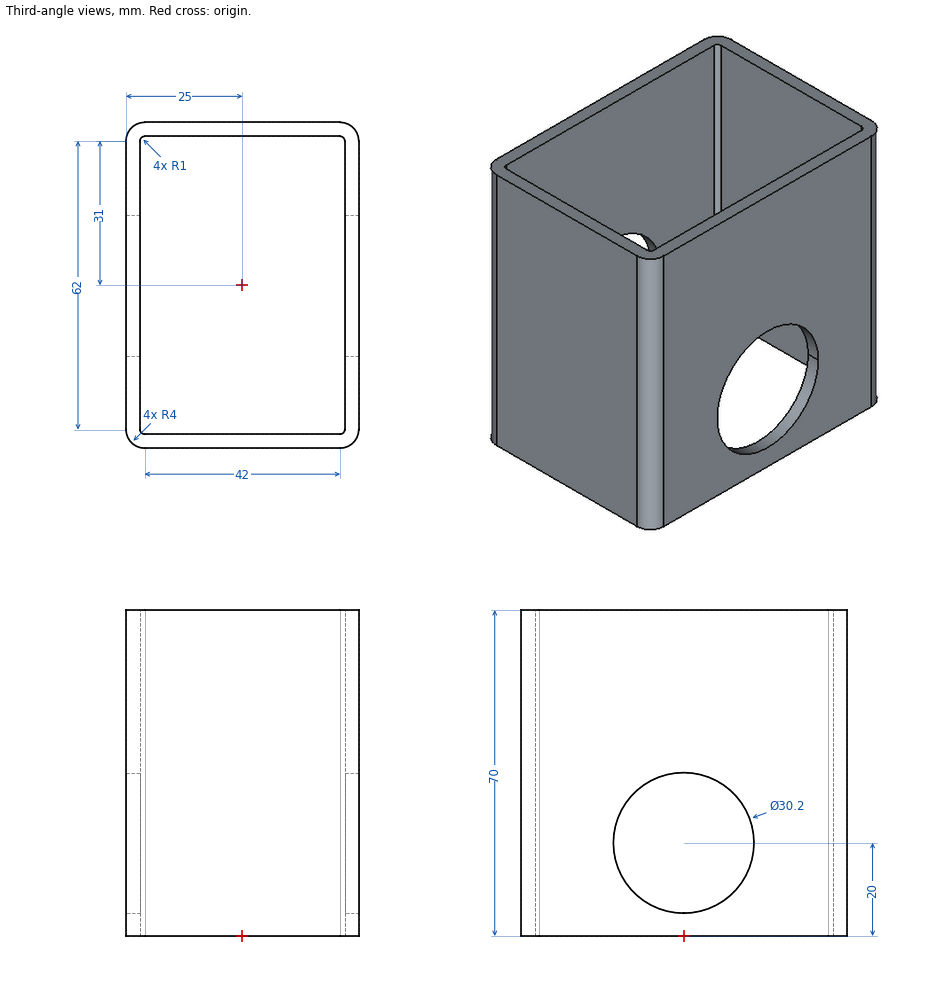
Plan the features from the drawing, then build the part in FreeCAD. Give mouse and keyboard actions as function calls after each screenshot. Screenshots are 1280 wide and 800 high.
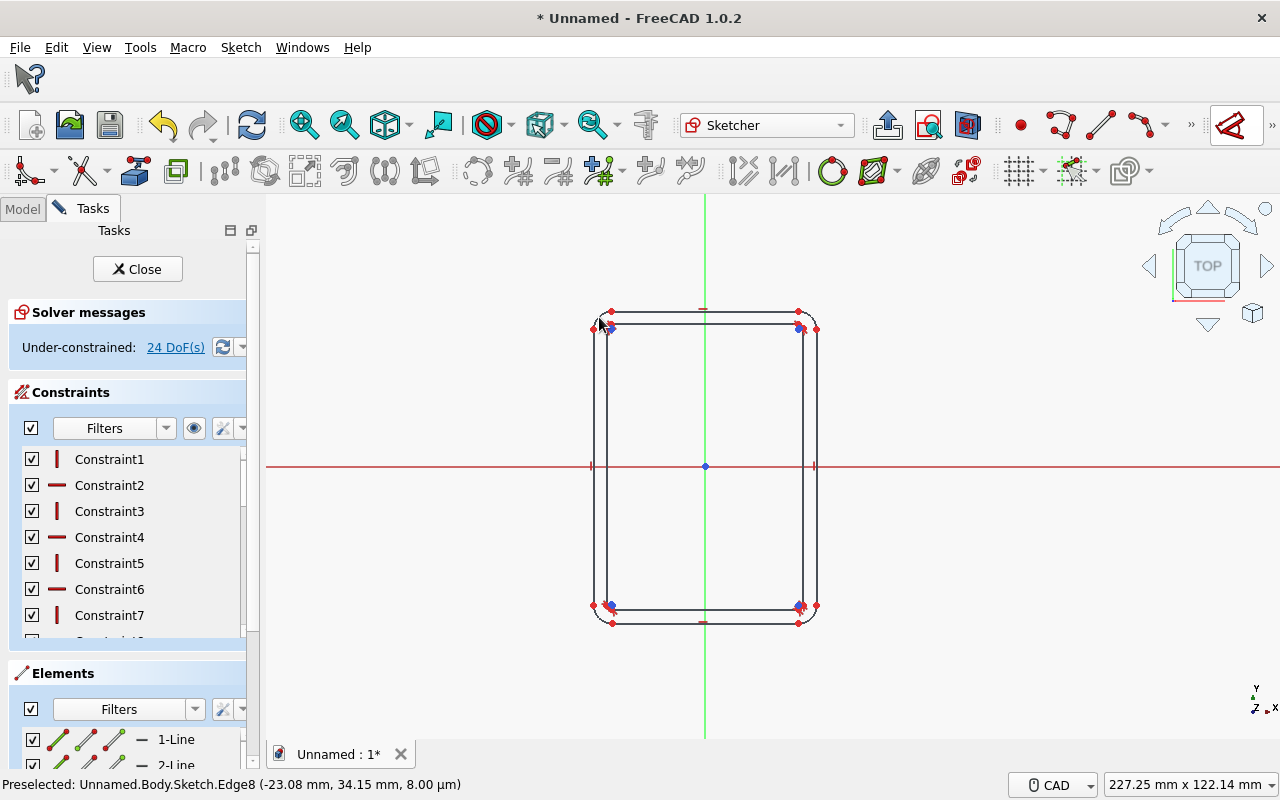
click(607, 522)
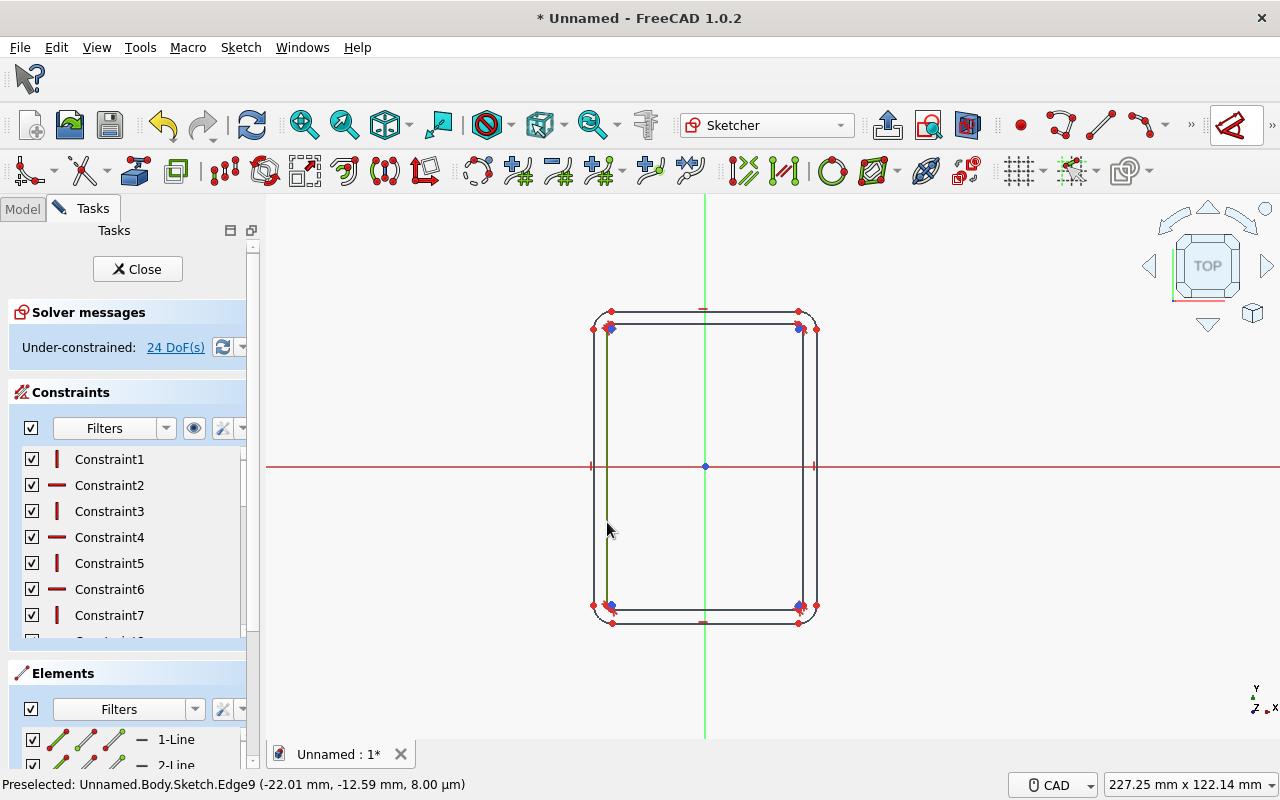
scroll(608, 326, up, 7)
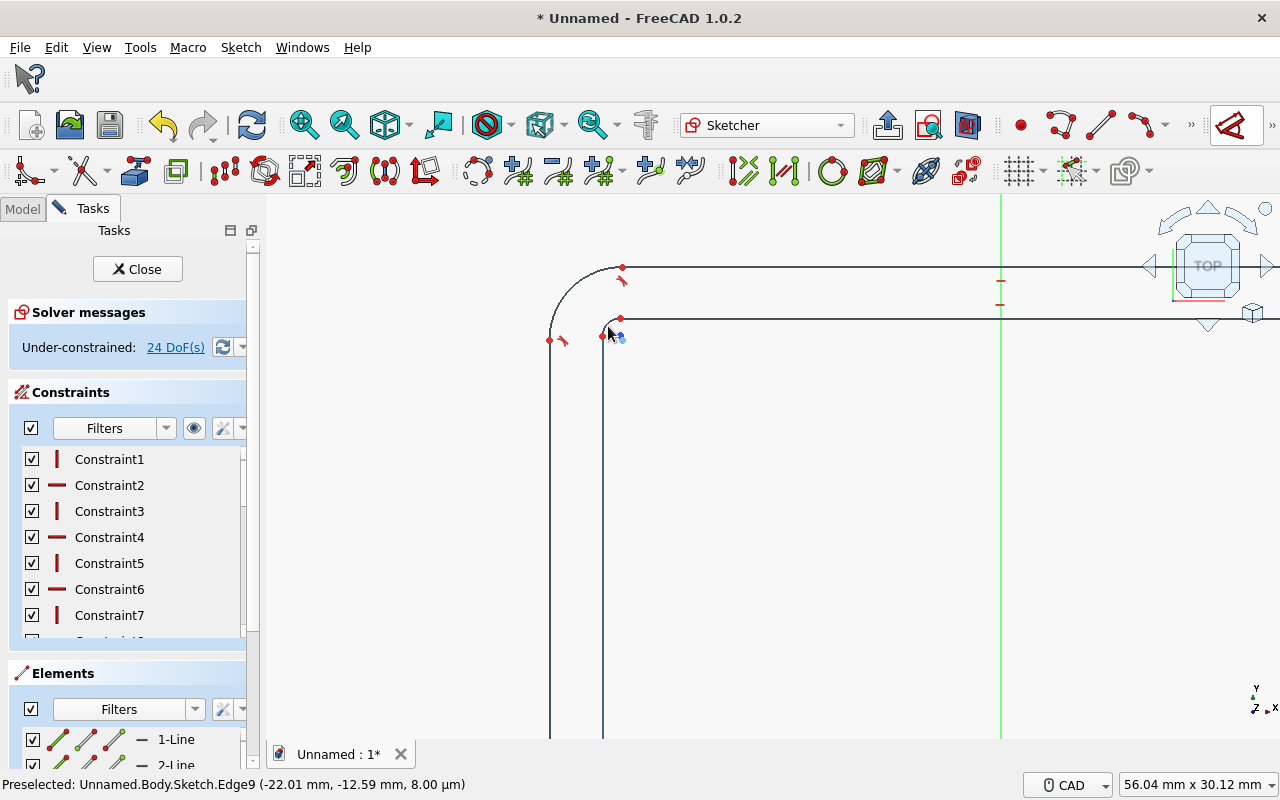
click(608, 324)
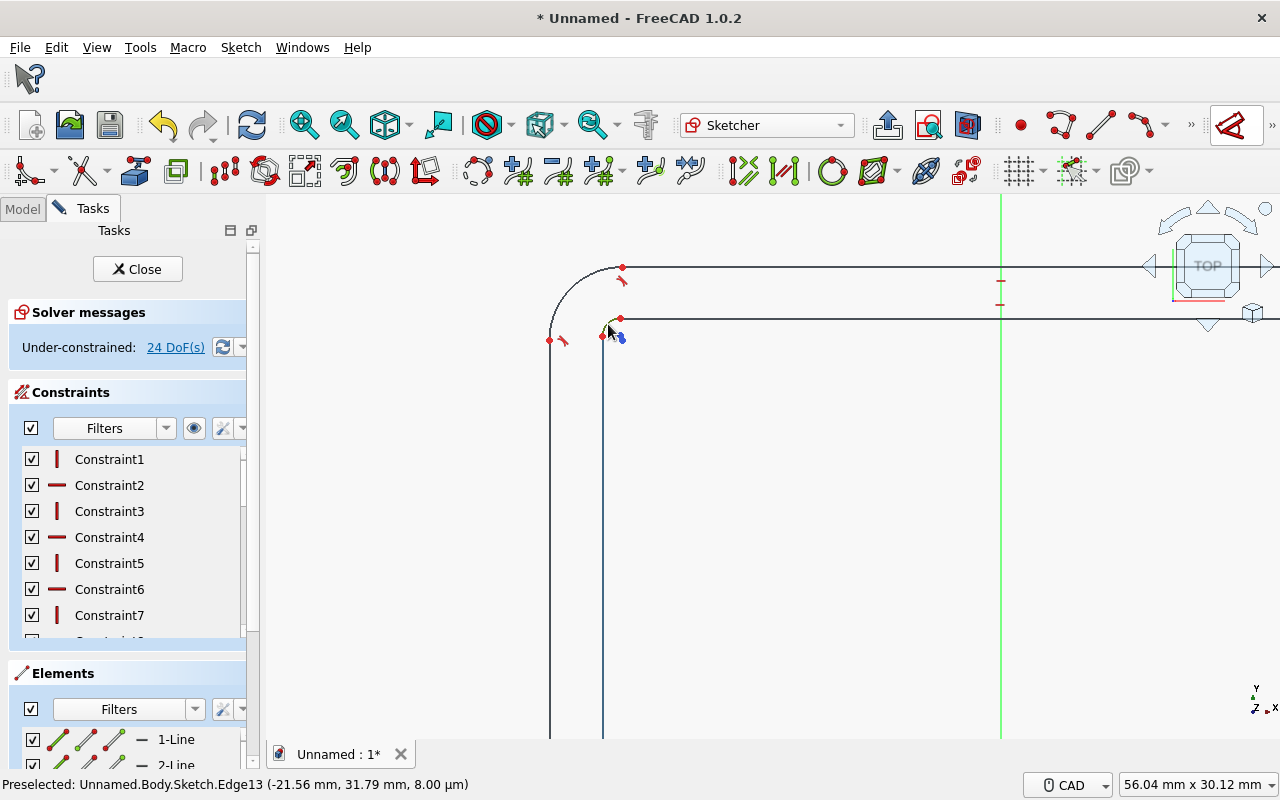
key(t)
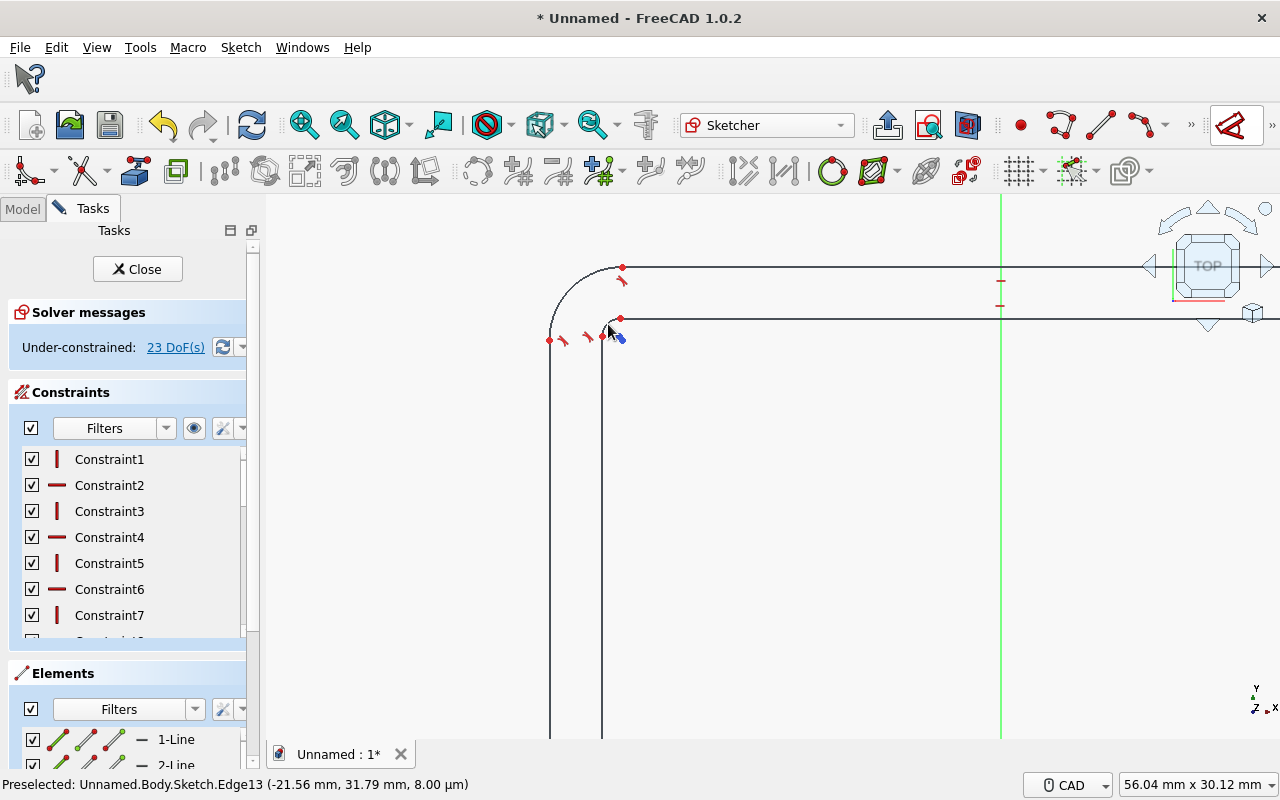
click(602, 673)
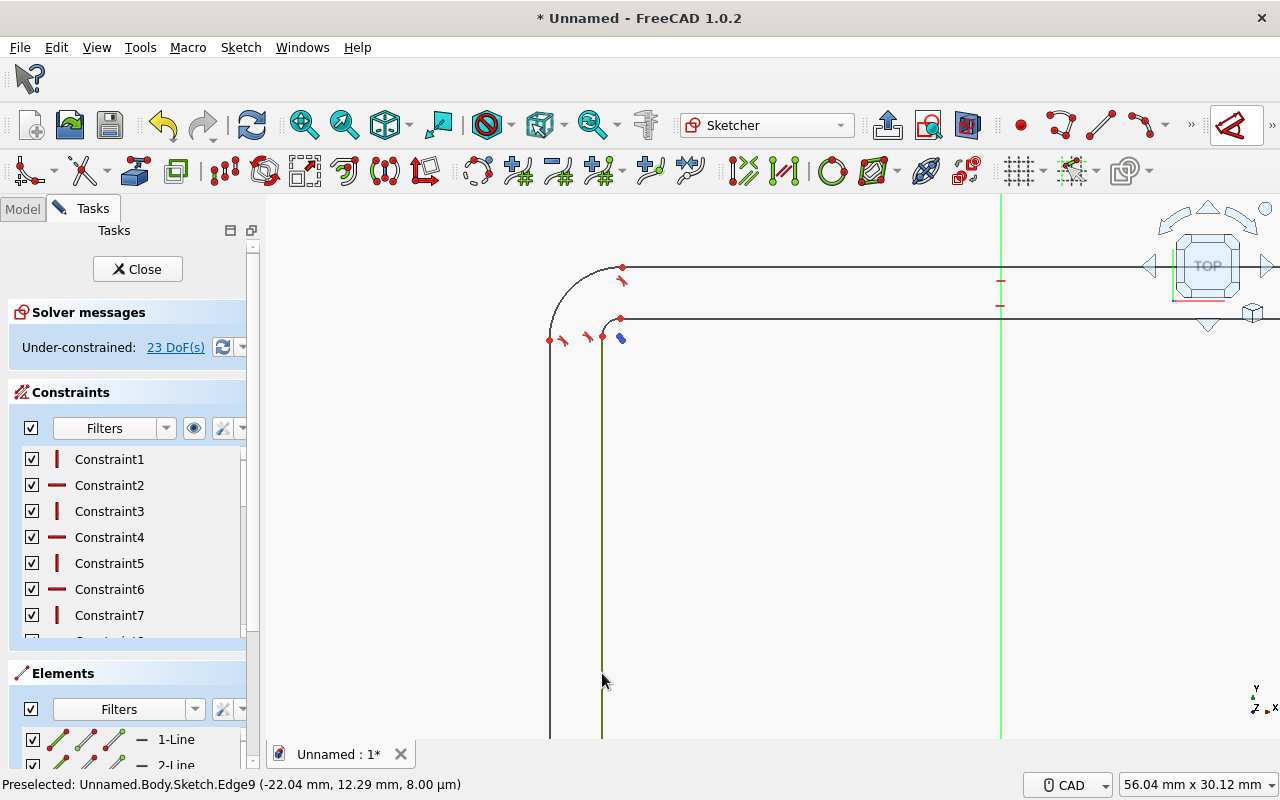
scroll(607, 326, down, 7)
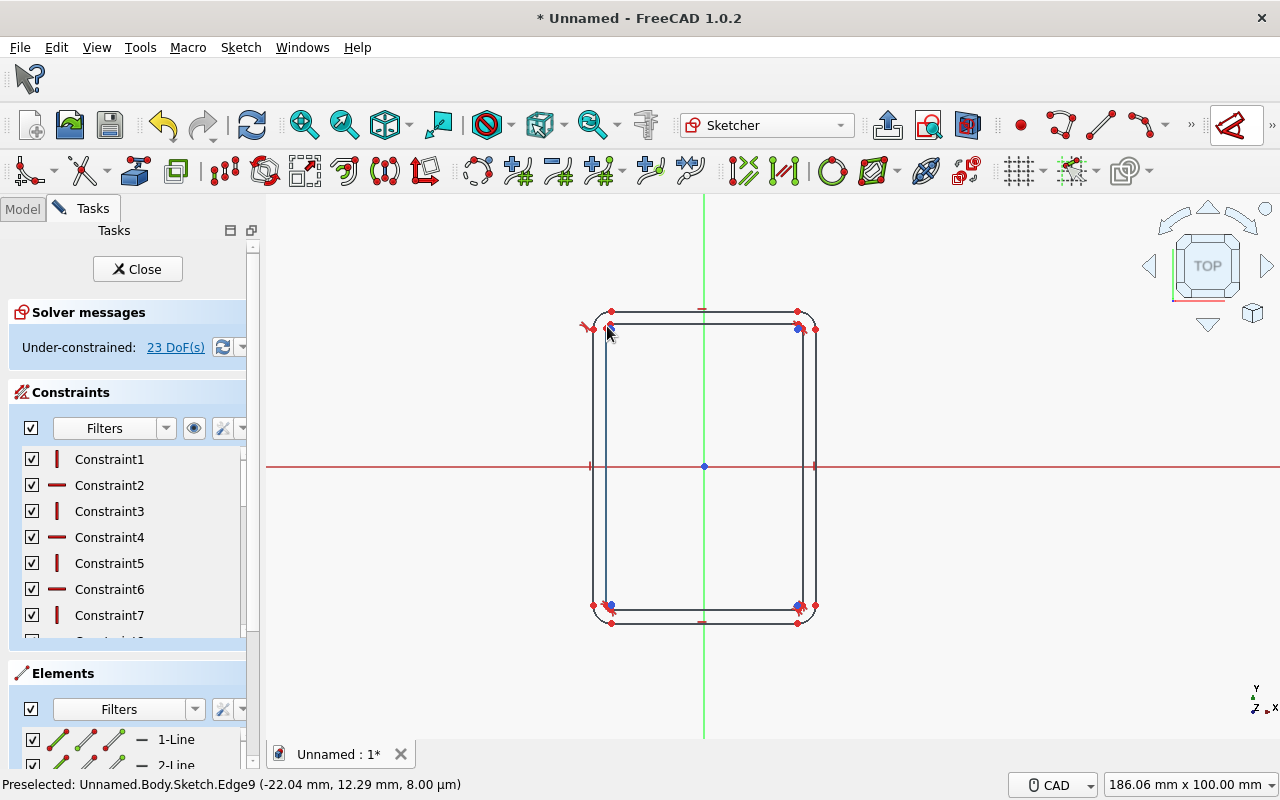
scroll(608, 609, up, 7)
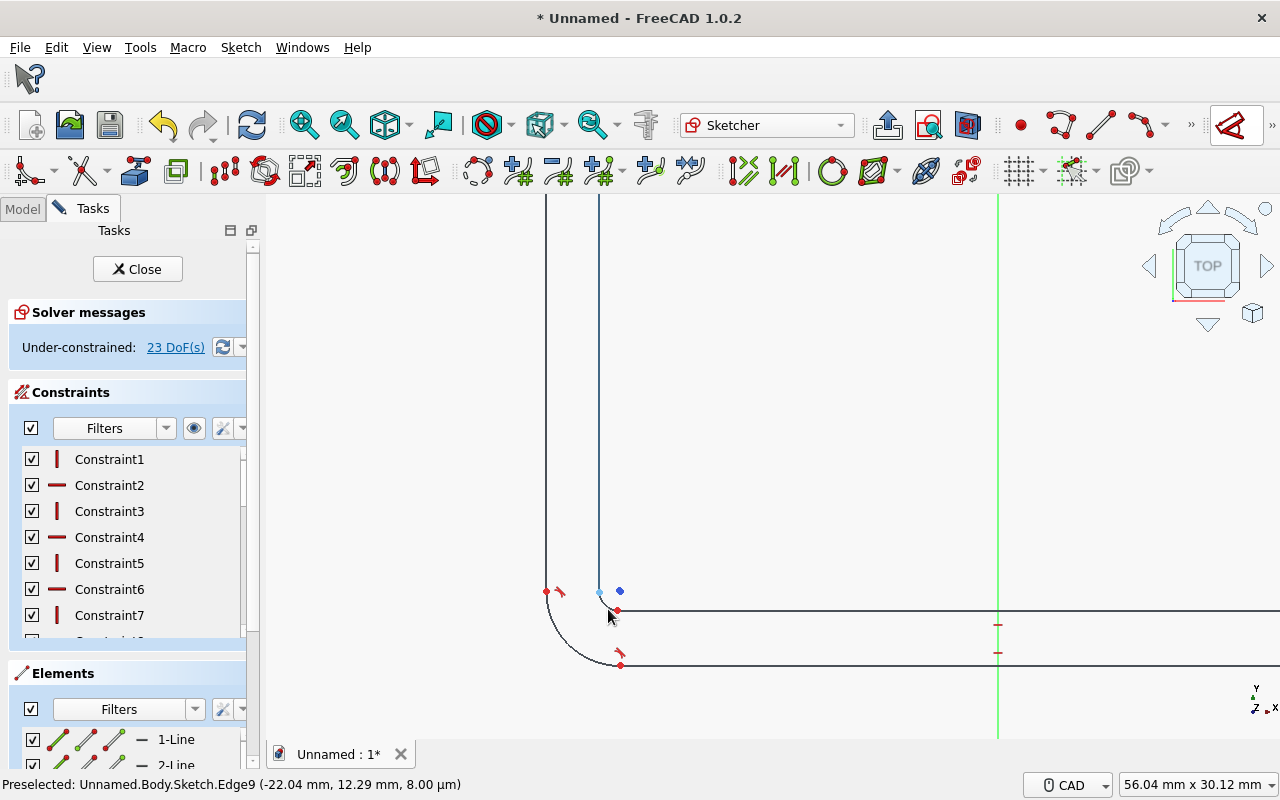
click(605, 605)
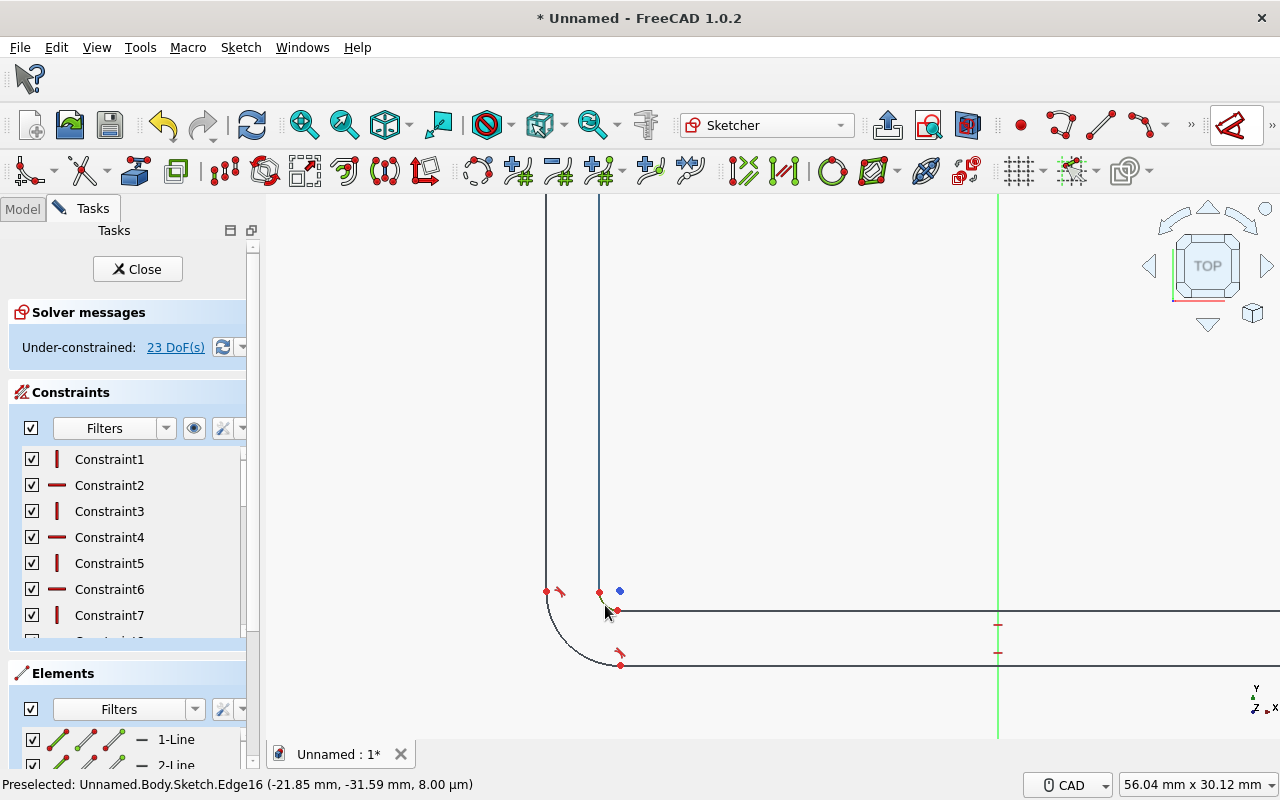
key(t)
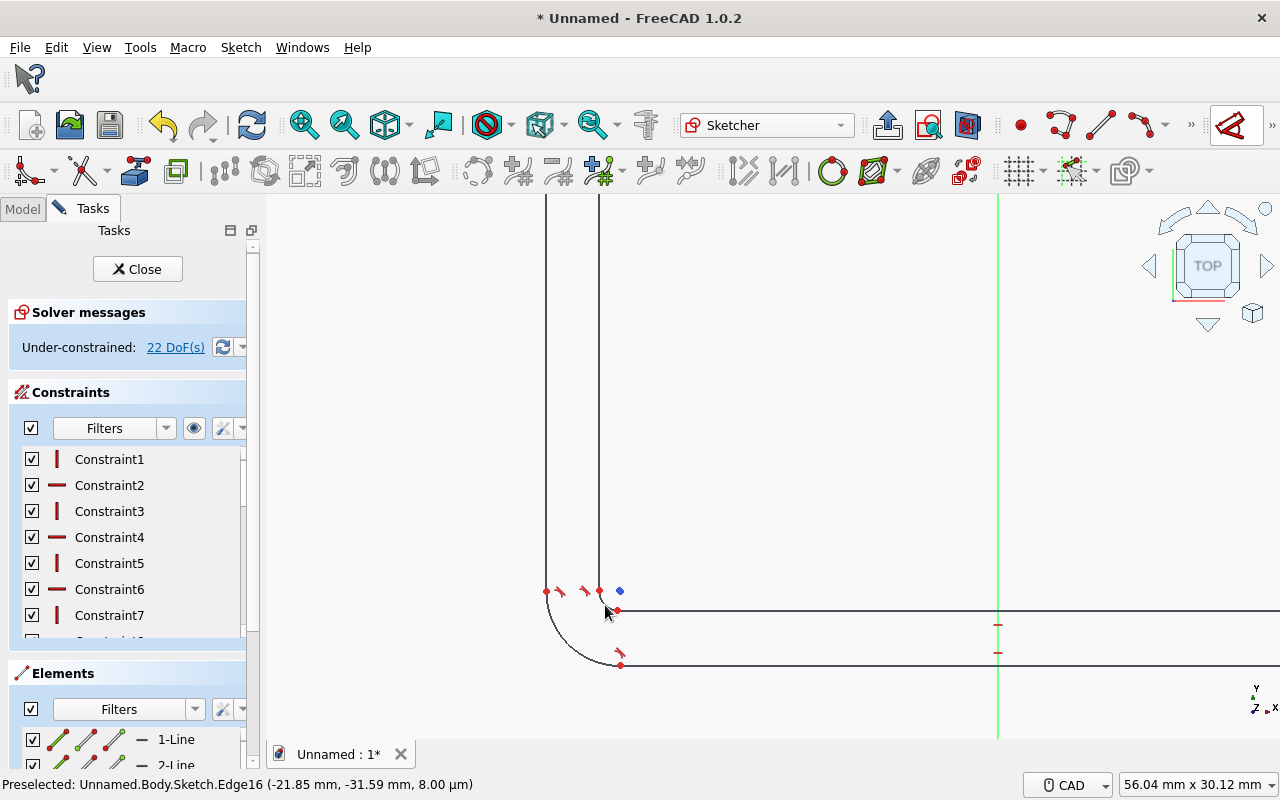
scroll(608, 609, down, 7)